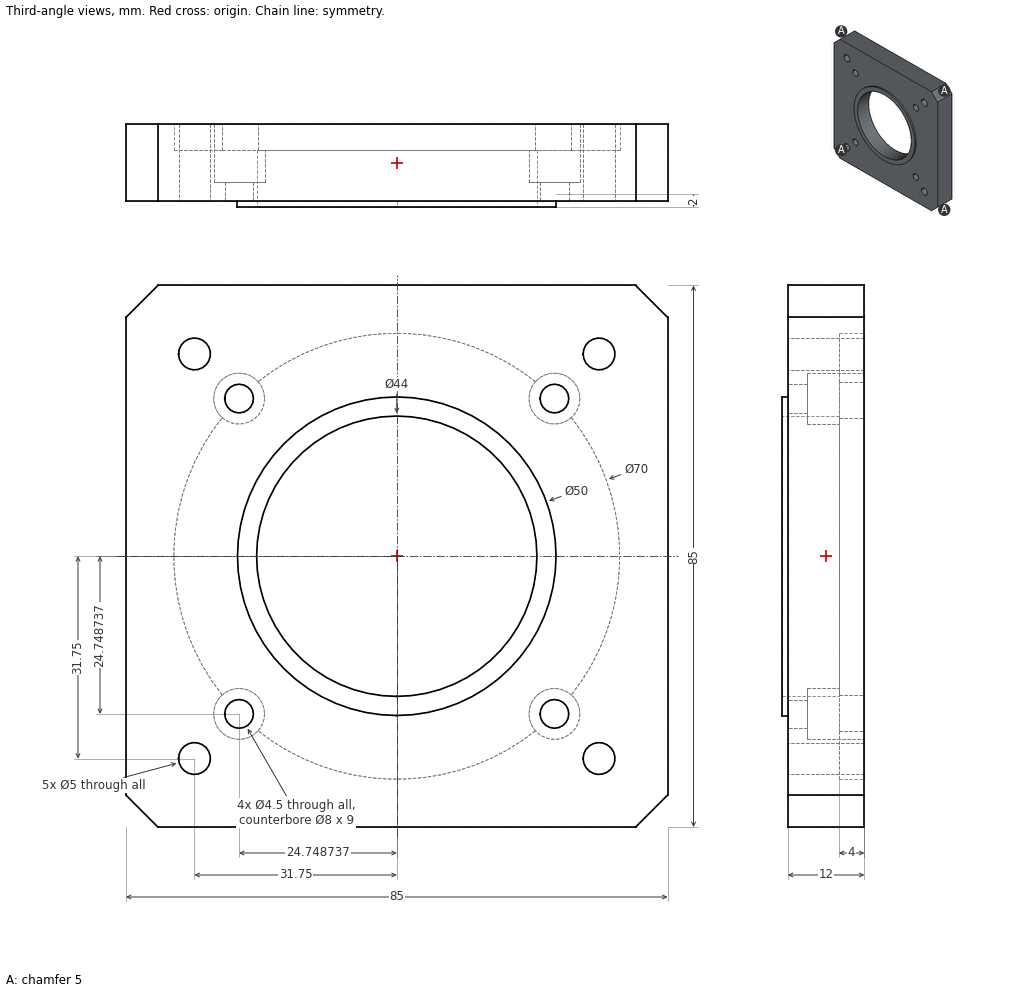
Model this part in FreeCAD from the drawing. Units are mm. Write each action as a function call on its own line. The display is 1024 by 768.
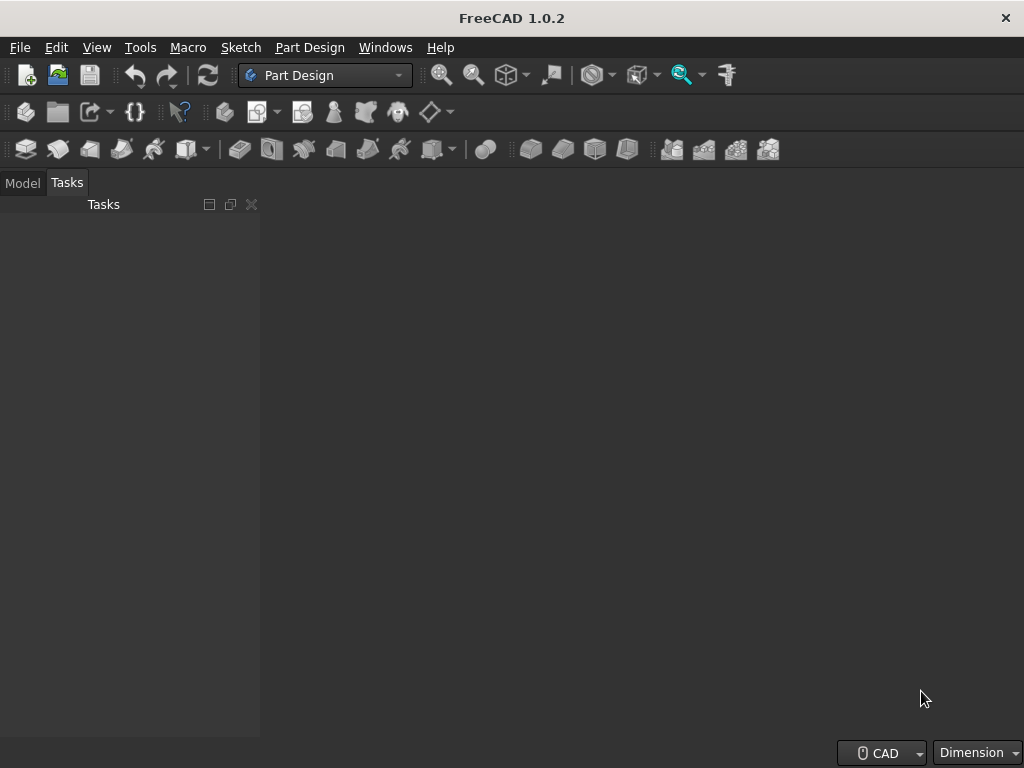
click(26, 76)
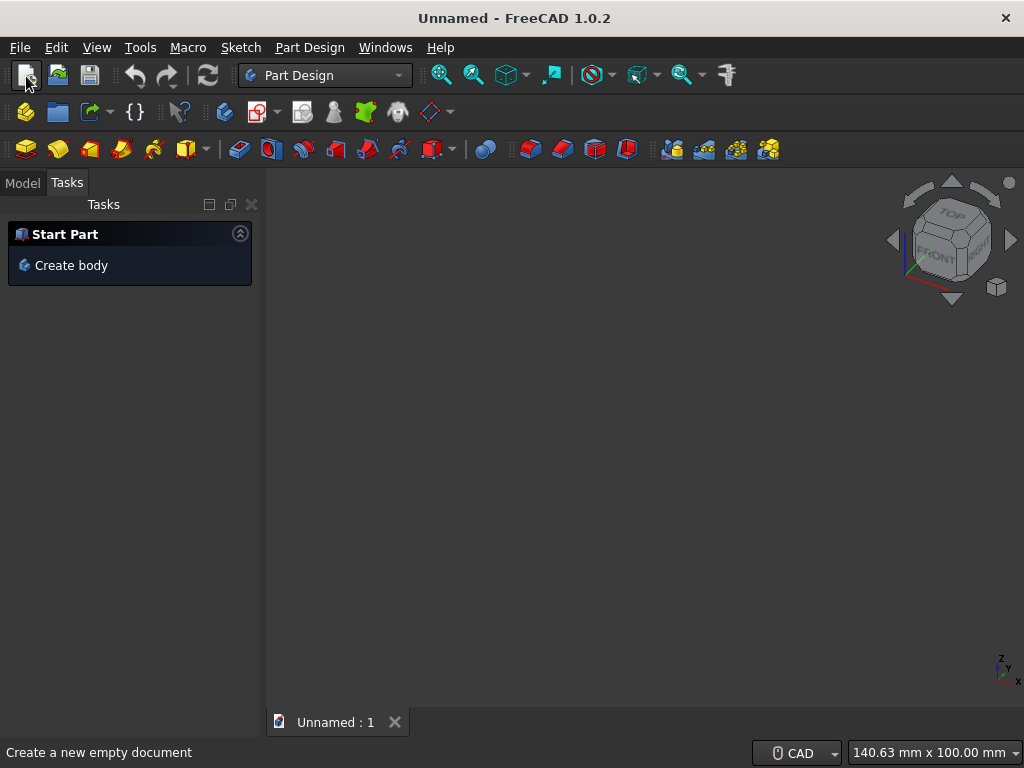
click(258, 112)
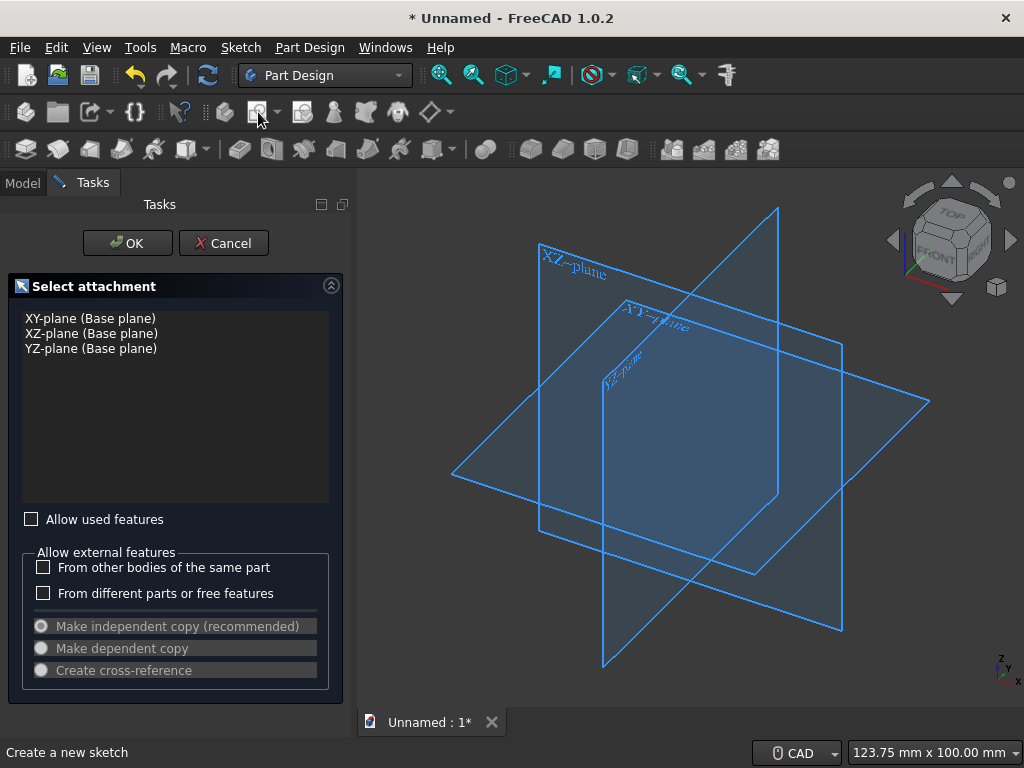
click(82, 334)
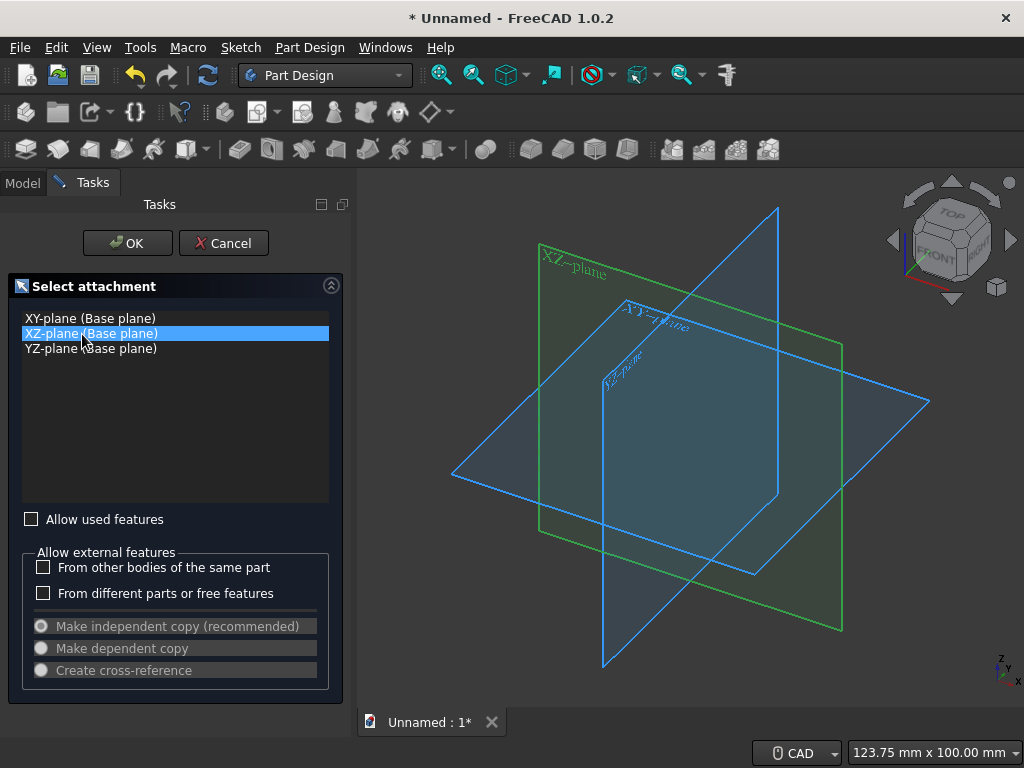
click(128, 243)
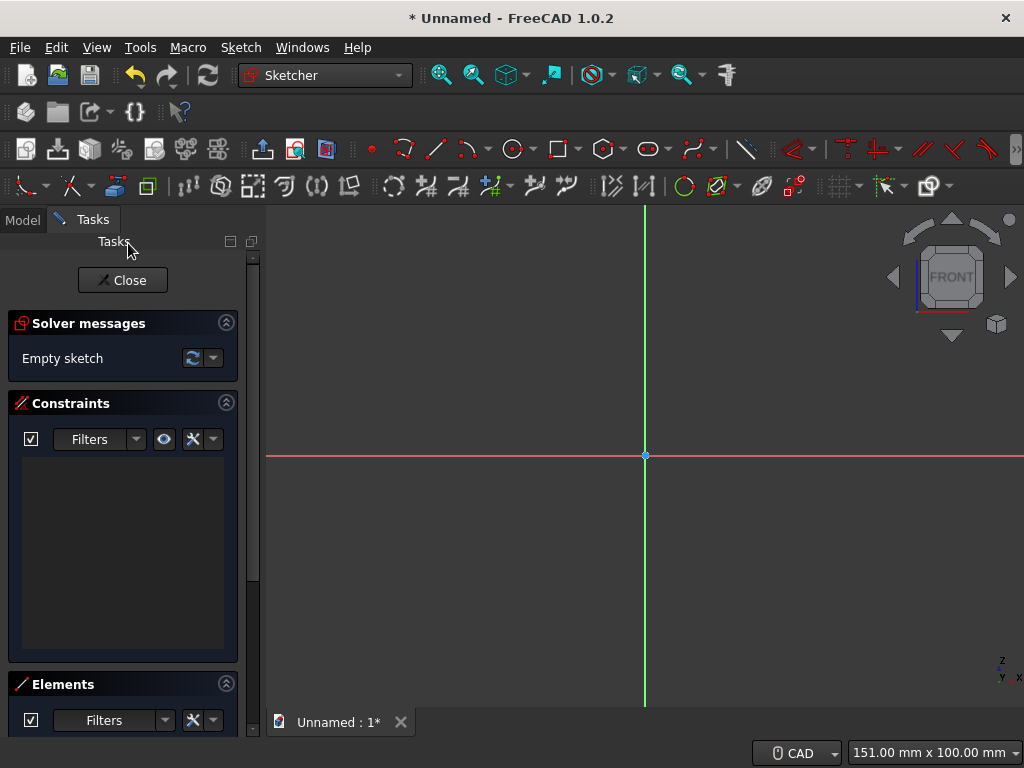
scroll(437, 456, down, 2)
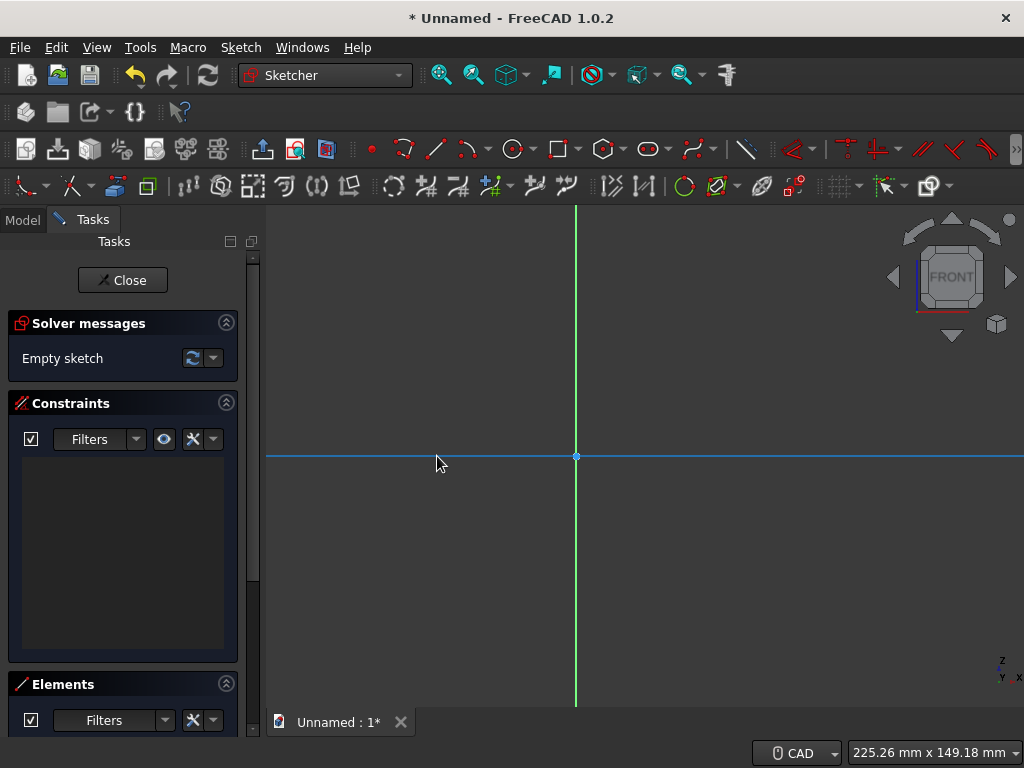
key(g)
key(v)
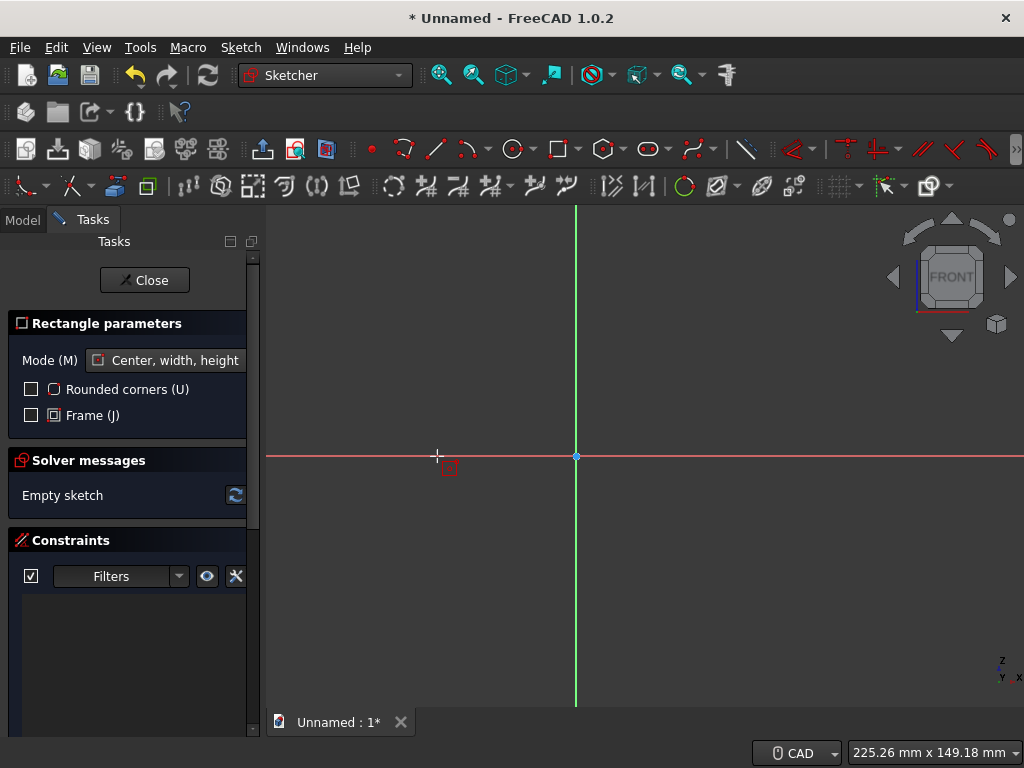
click(577, 456)
move(720, 313)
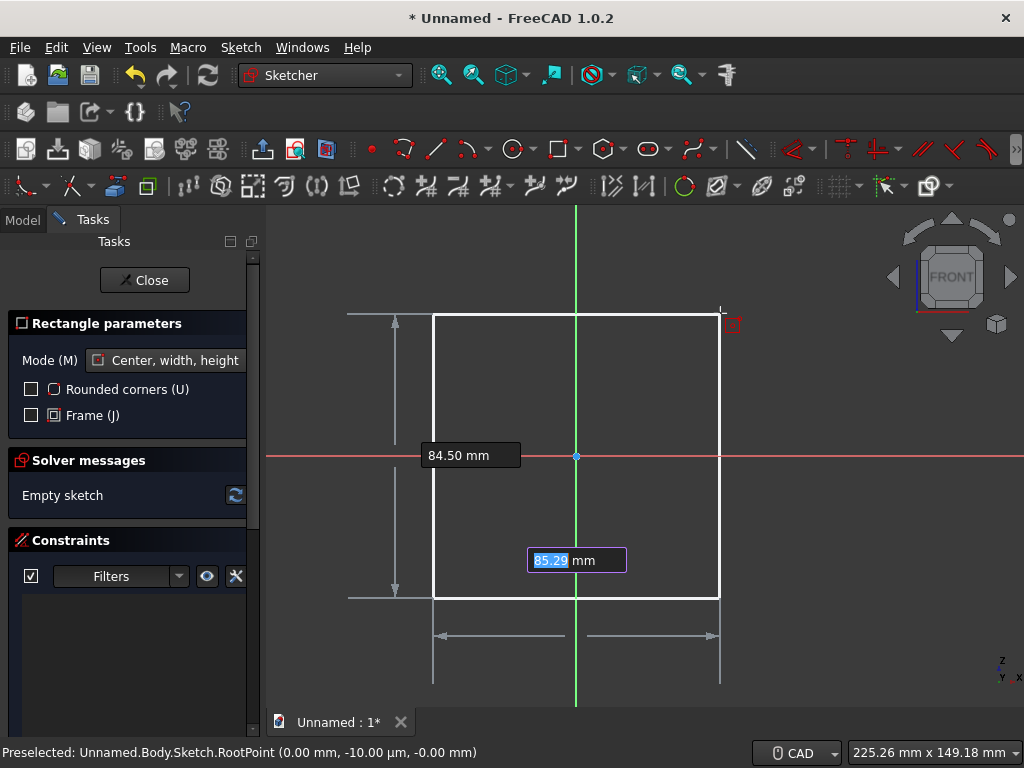
text(85)
key(Tab)
text(85)
key(Return)
key(Escape)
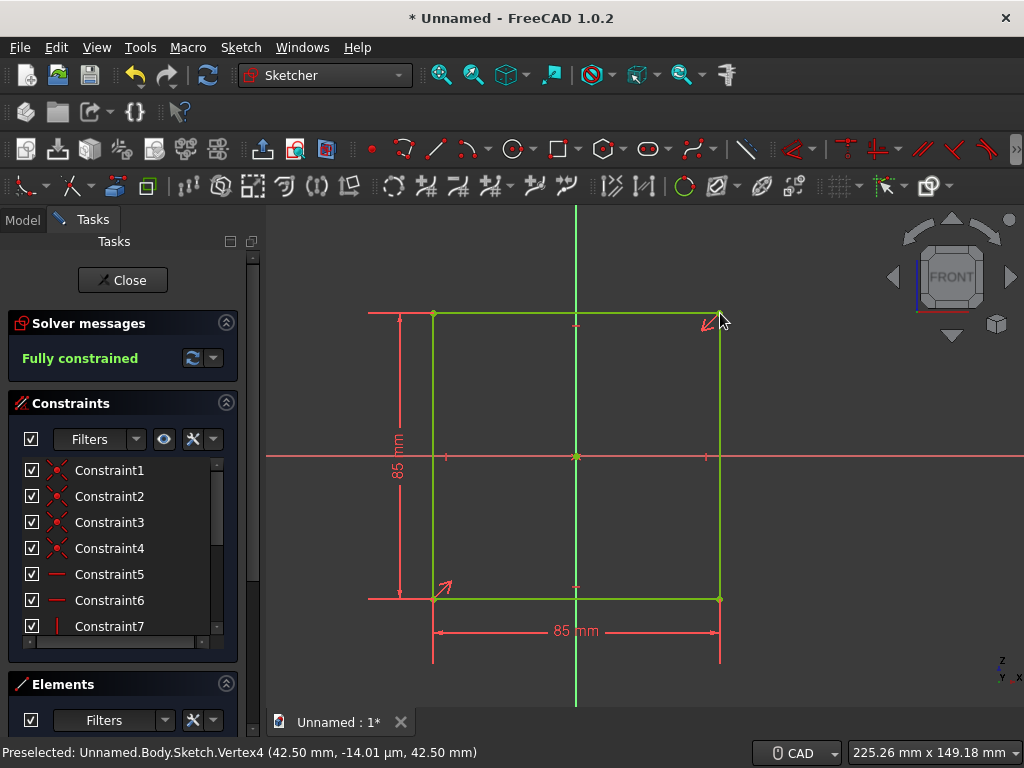
click(123, 280)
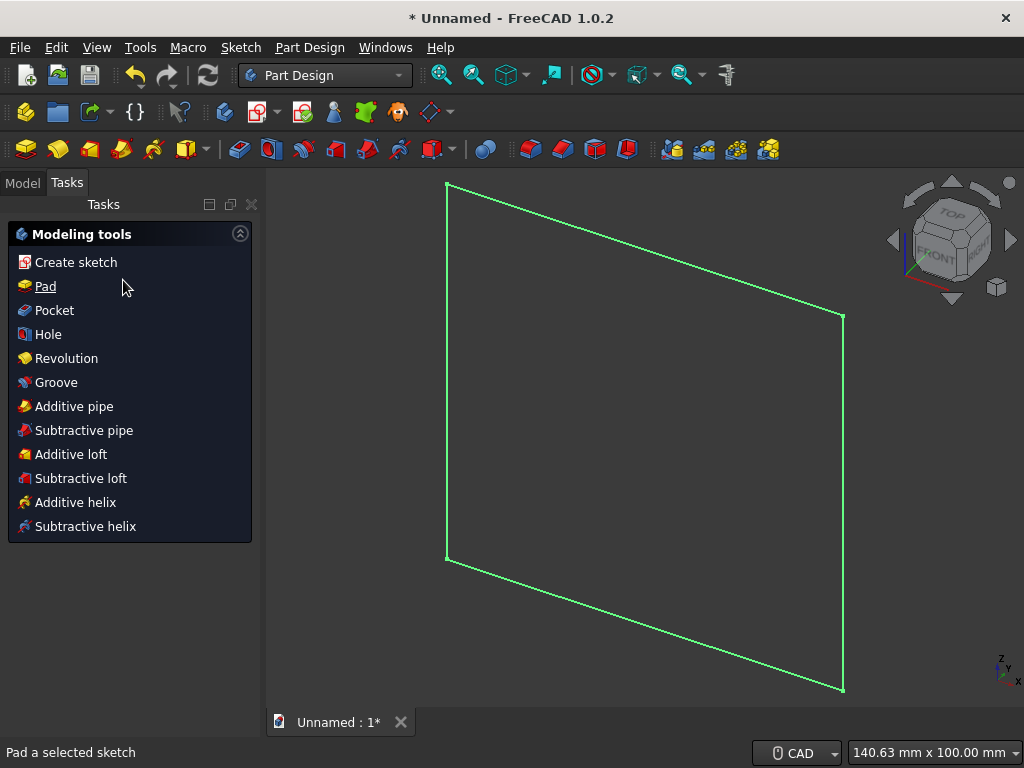
click(26, 150)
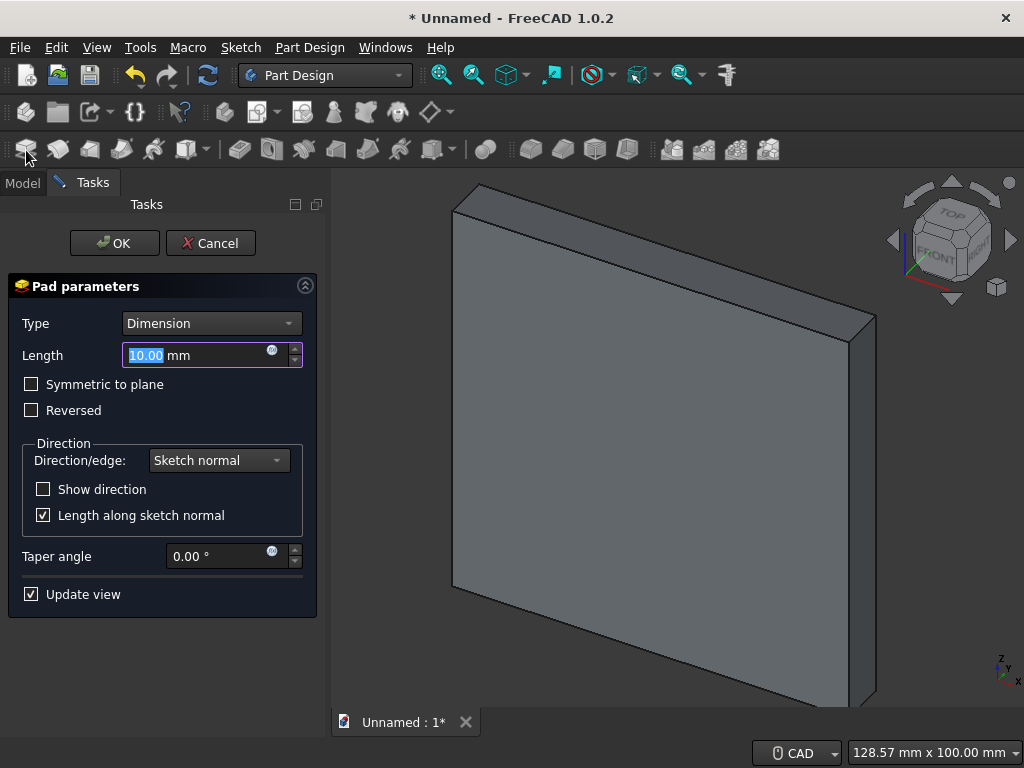
text(12)
key(Tab)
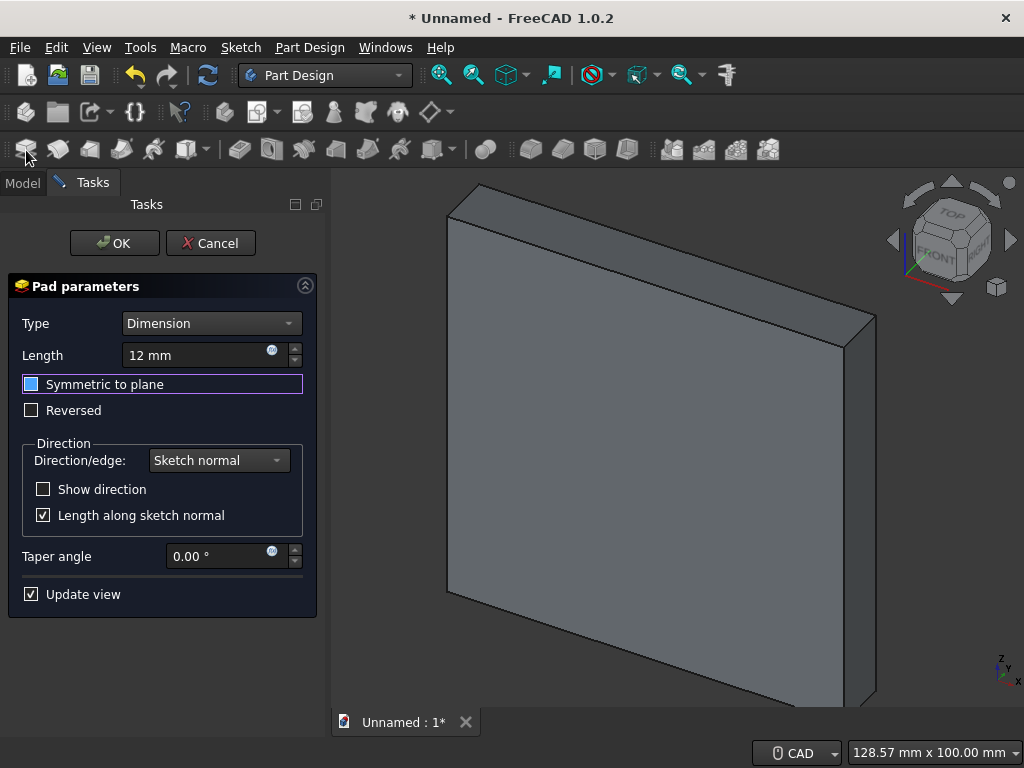
click(30, 384)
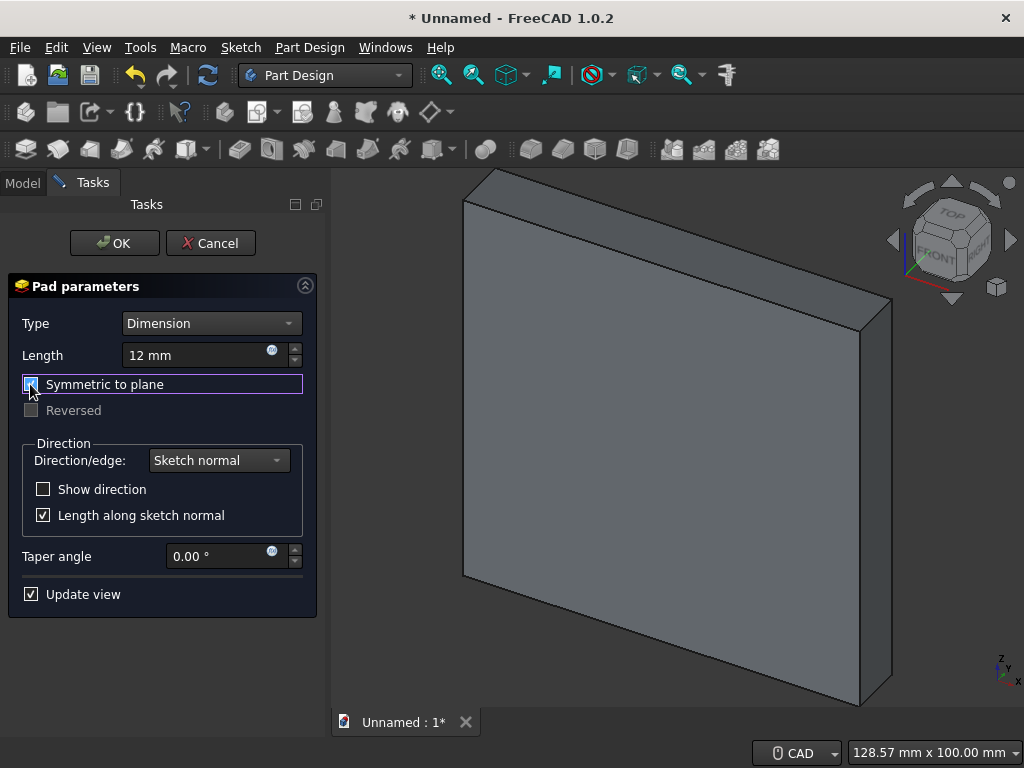
click(115, 243)